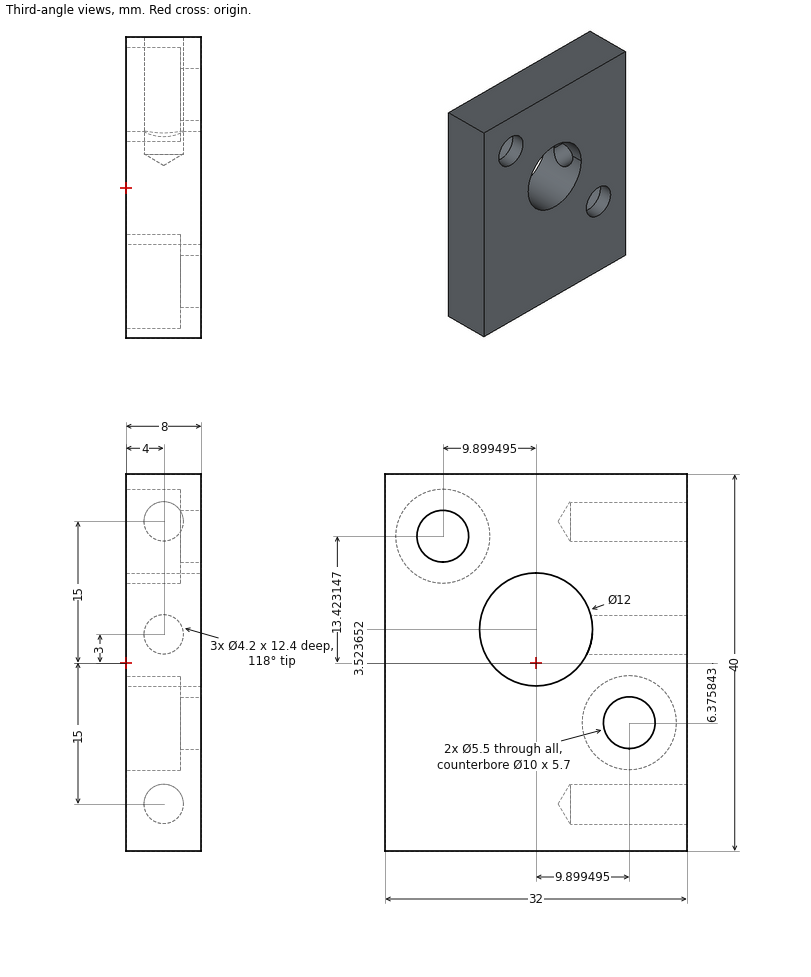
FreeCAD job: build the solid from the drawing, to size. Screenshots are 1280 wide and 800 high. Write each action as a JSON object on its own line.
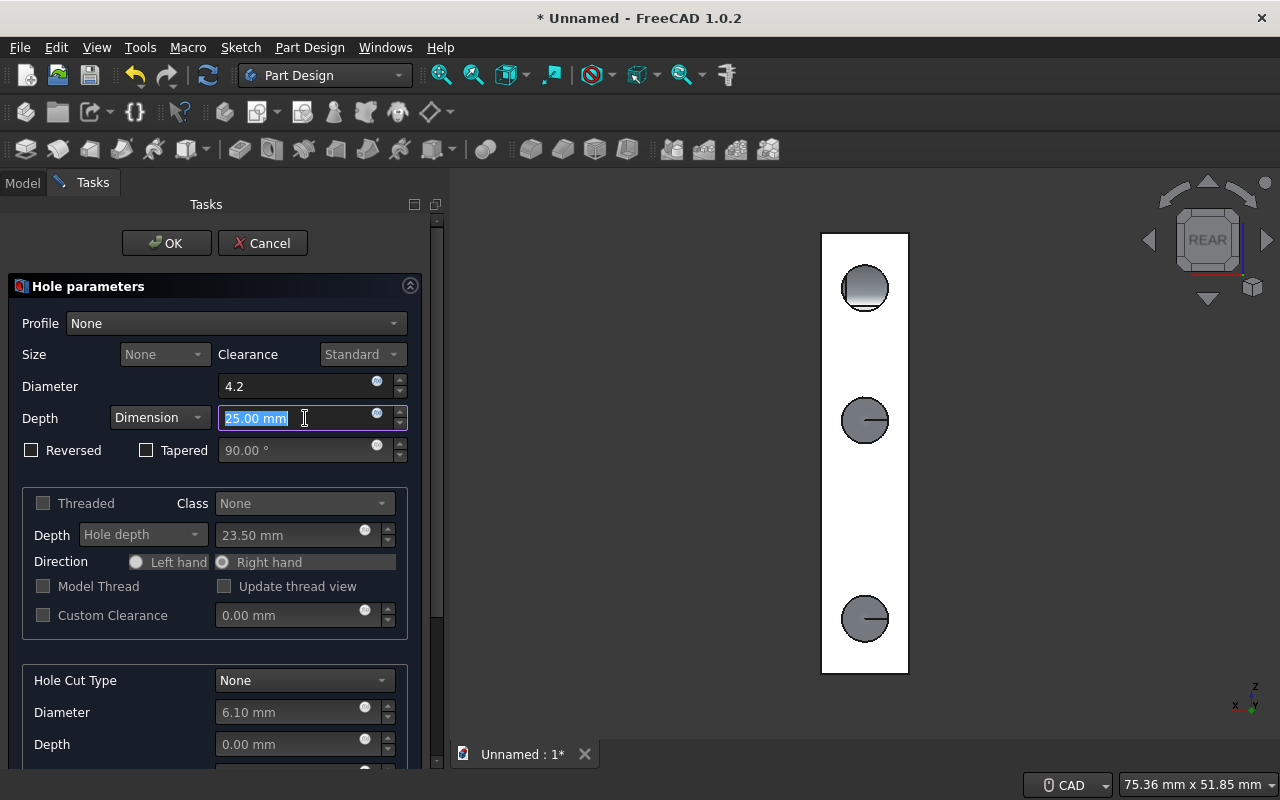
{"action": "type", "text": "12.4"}
{"action": "key", "text": "Tab"}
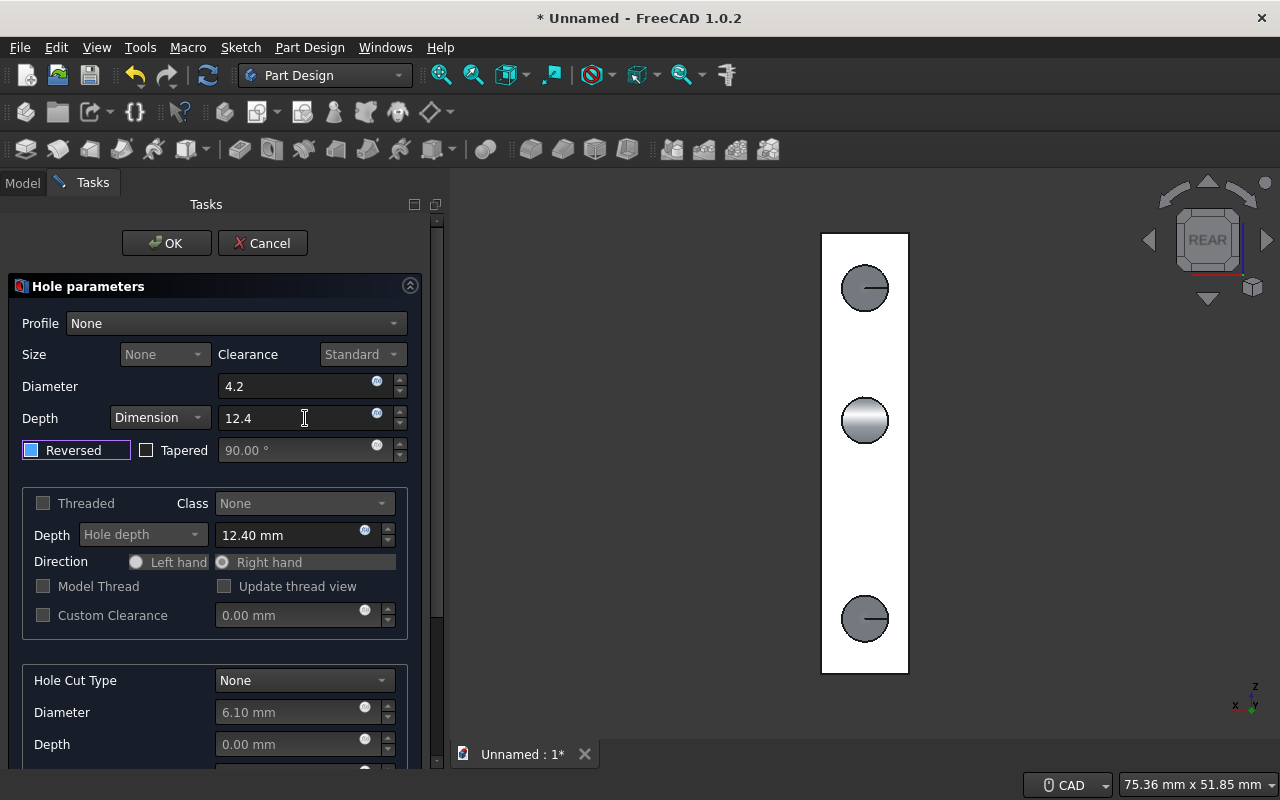
{"action": "left_click", "coordinate": [167, 243]}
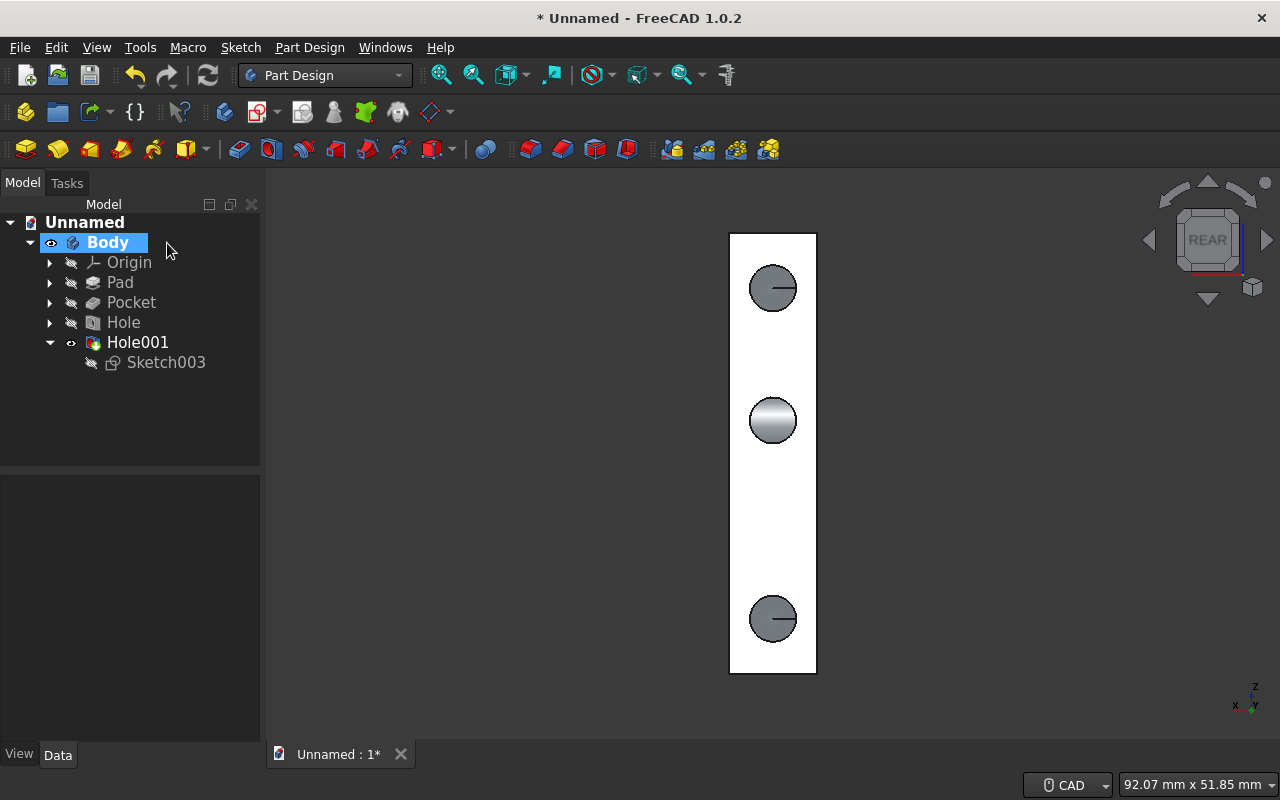
{"action": "key", "text": "0"}